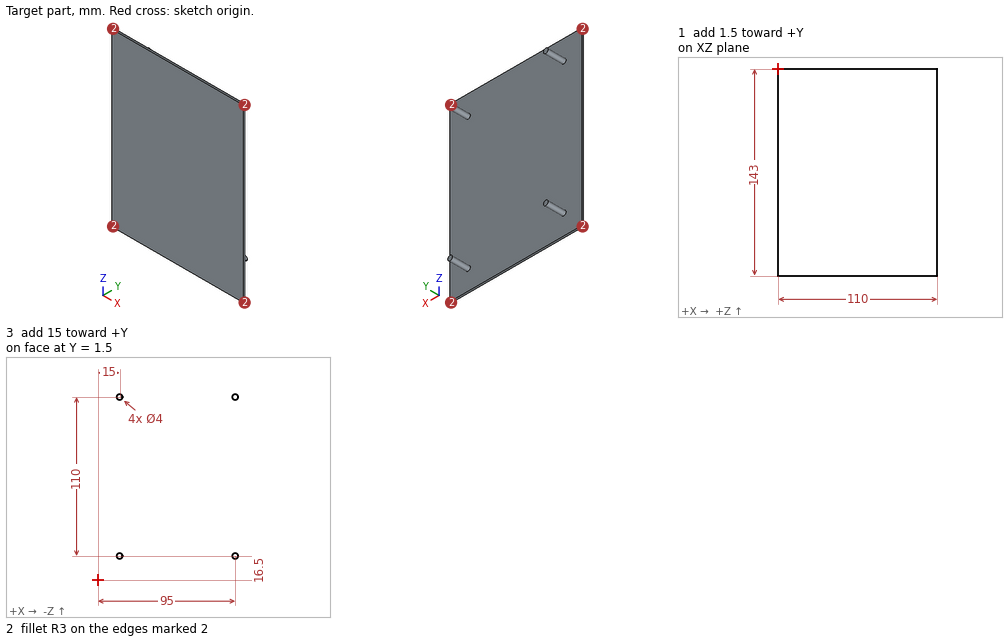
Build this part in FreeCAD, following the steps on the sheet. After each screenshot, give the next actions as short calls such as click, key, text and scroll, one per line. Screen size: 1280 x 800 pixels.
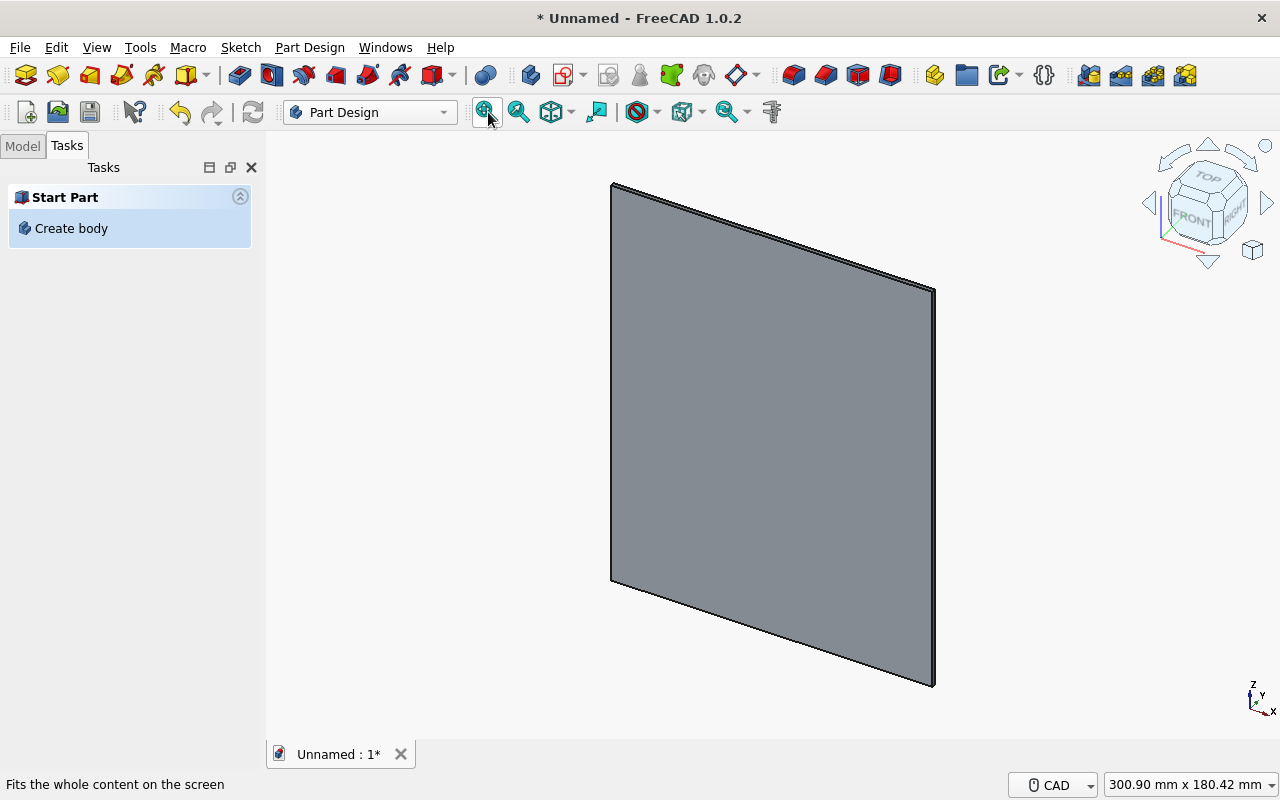
key(0)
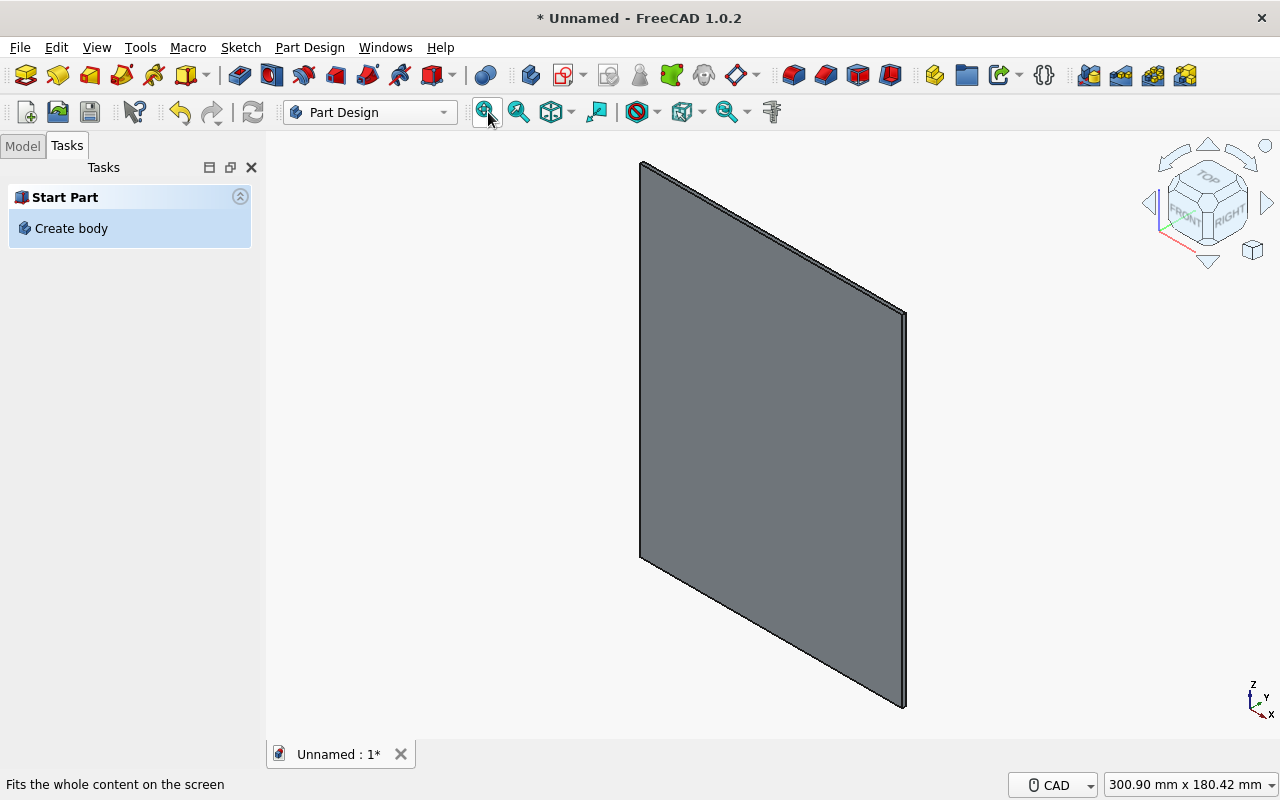
scroll(642, 555, up, 11)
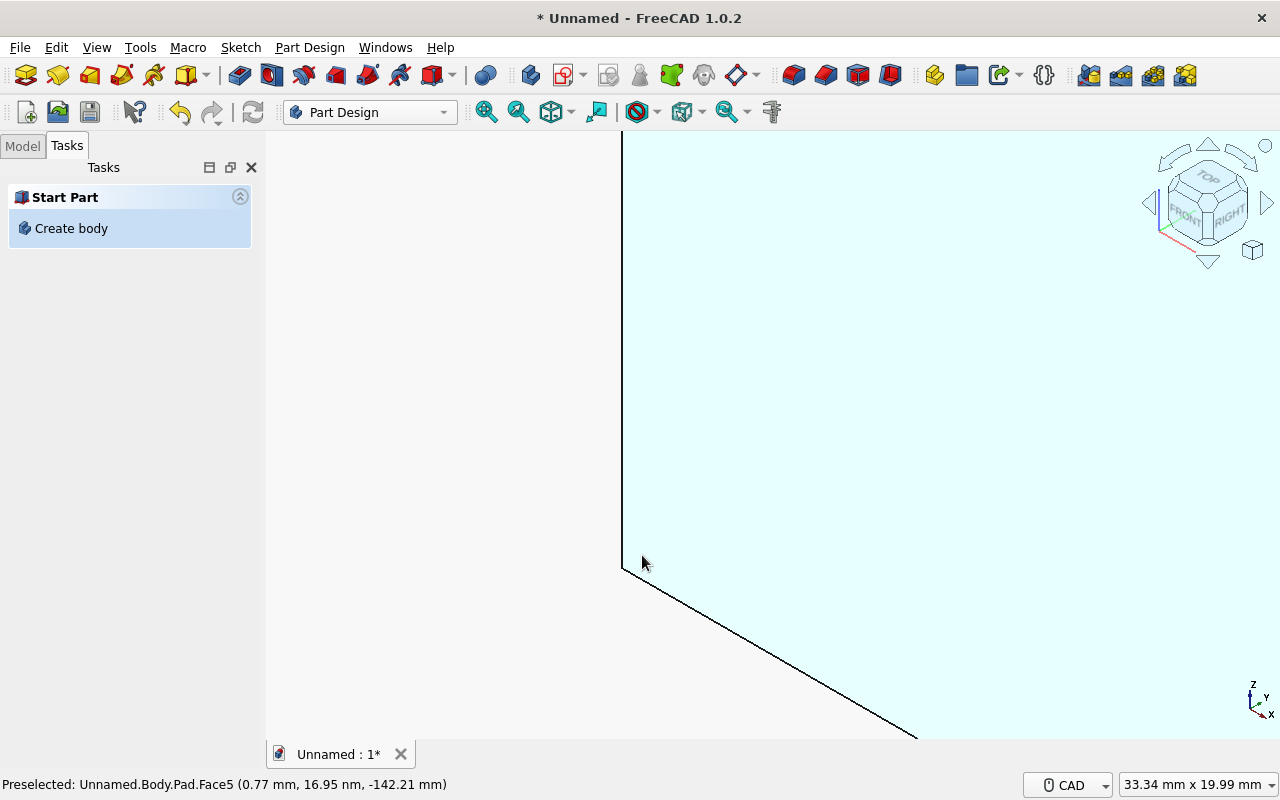
click(488, 112)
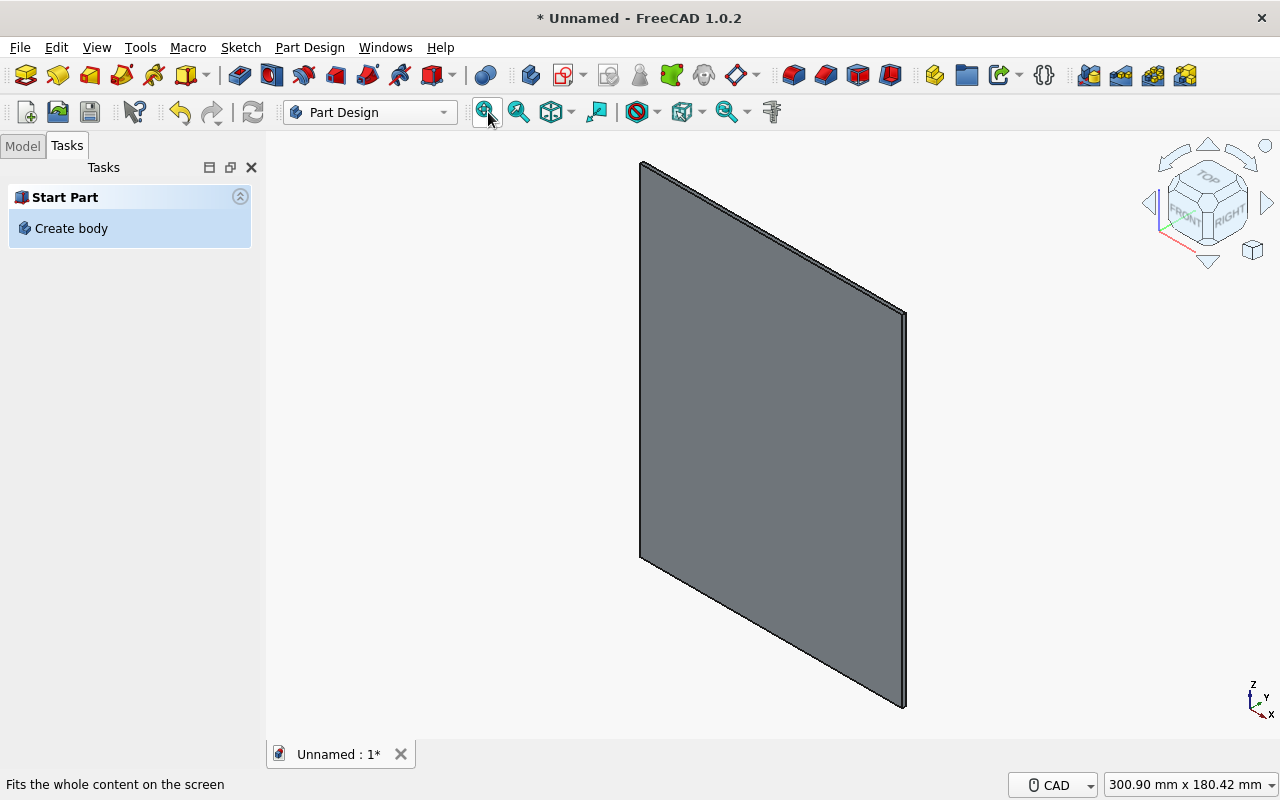
key(2)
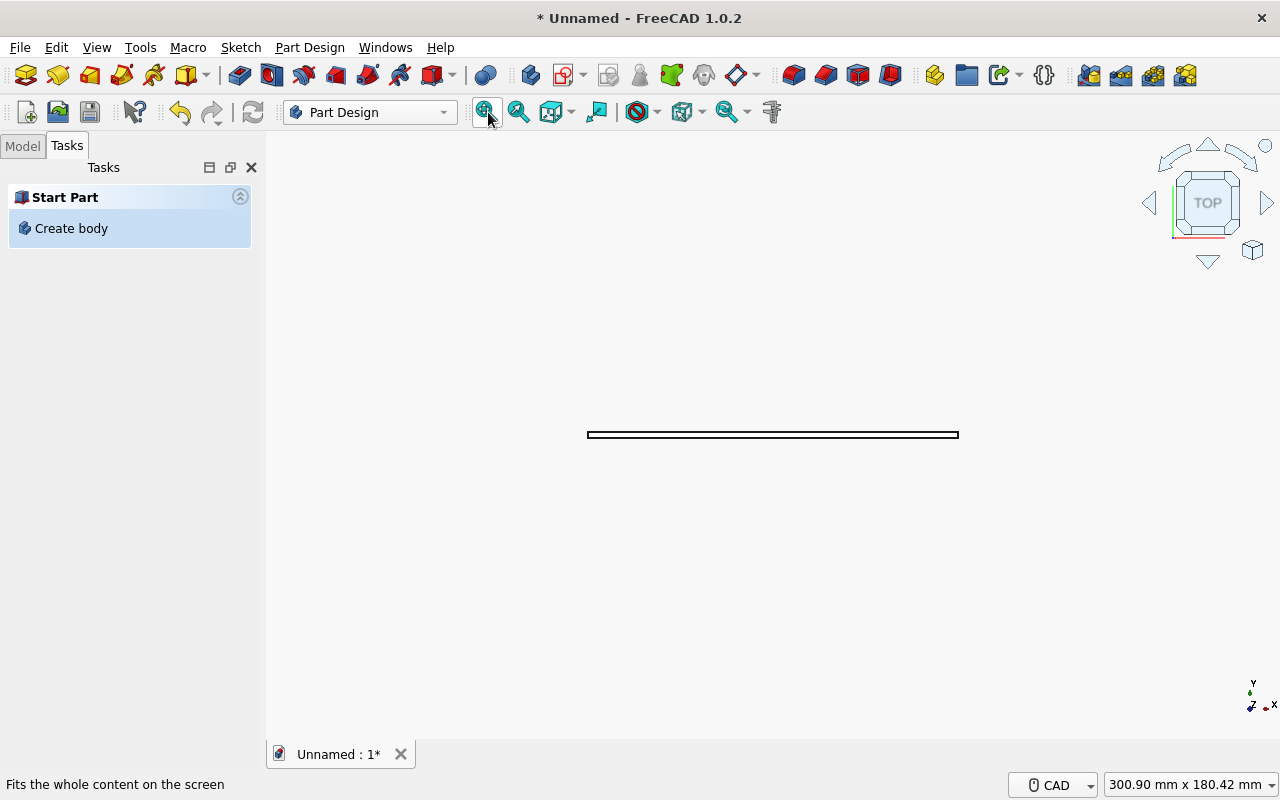
click(488, 112)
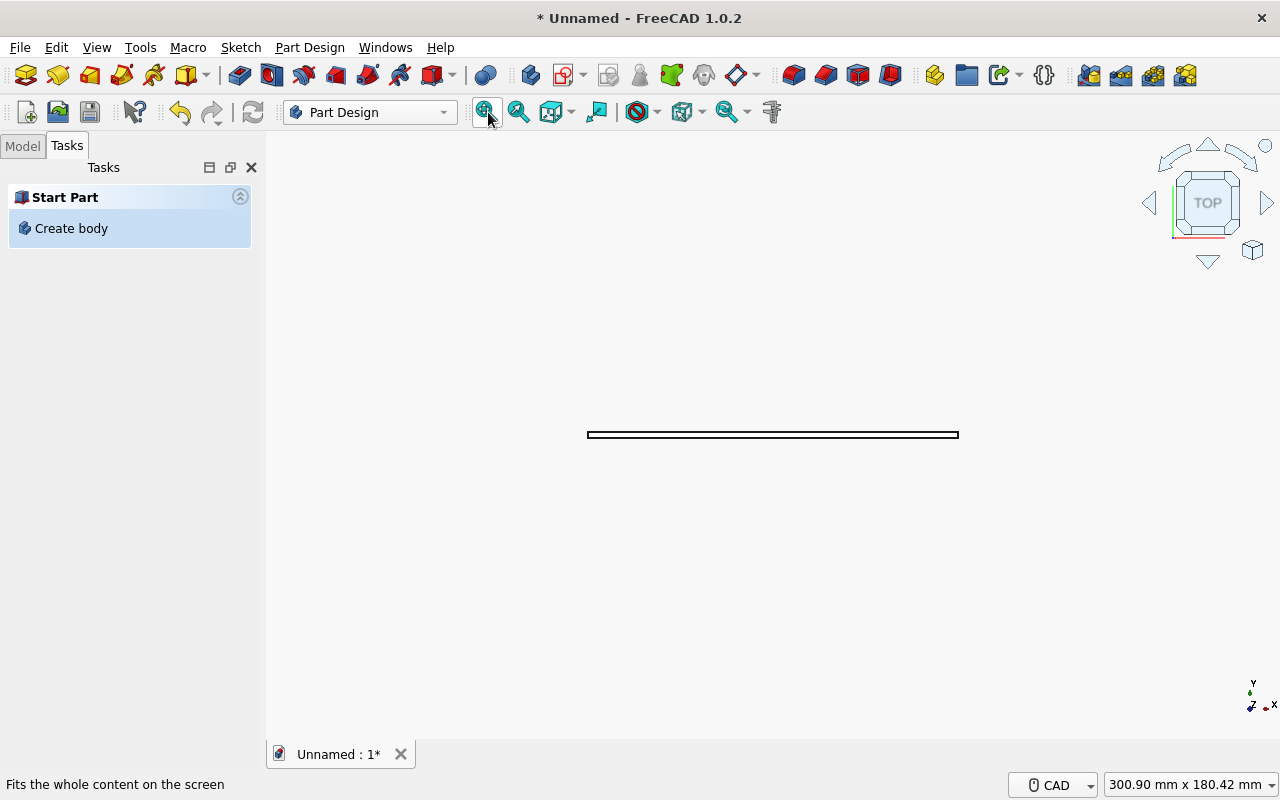
scroll(588, 434, up, 11)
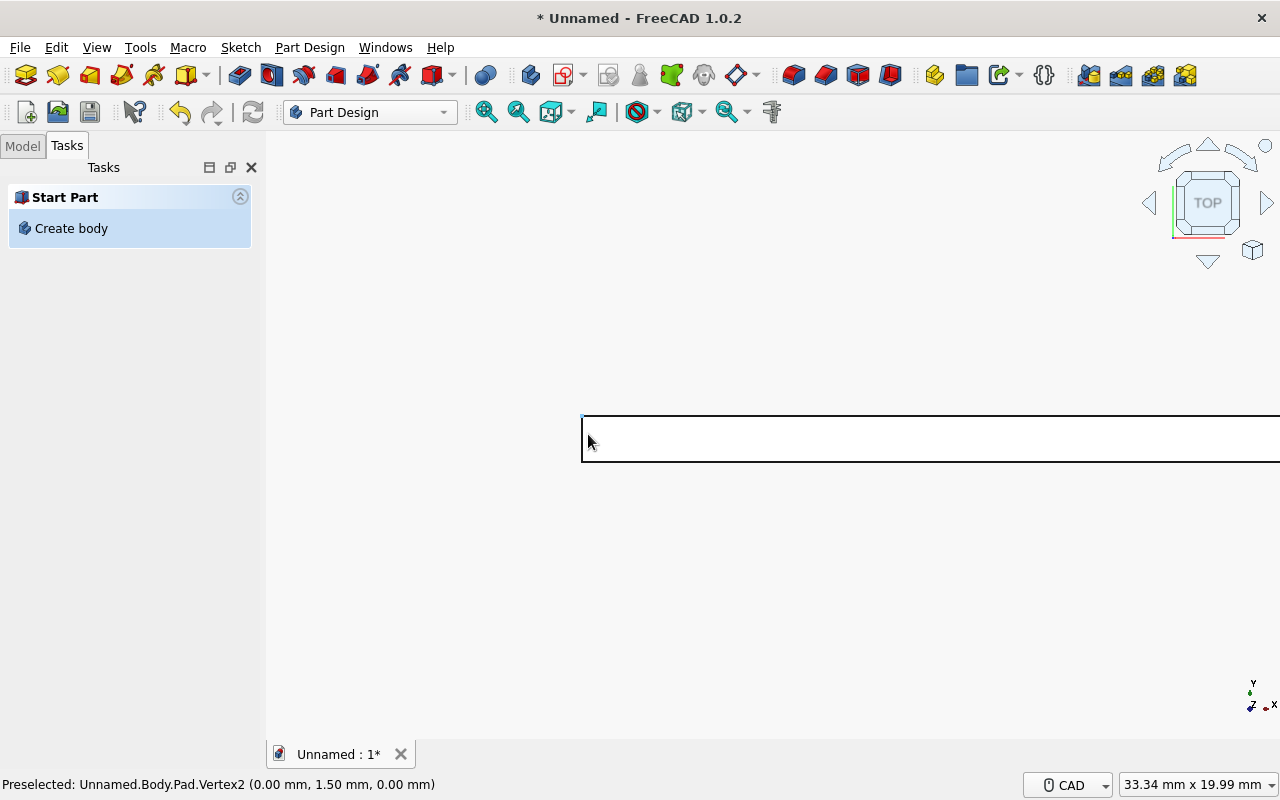
click(582, 438)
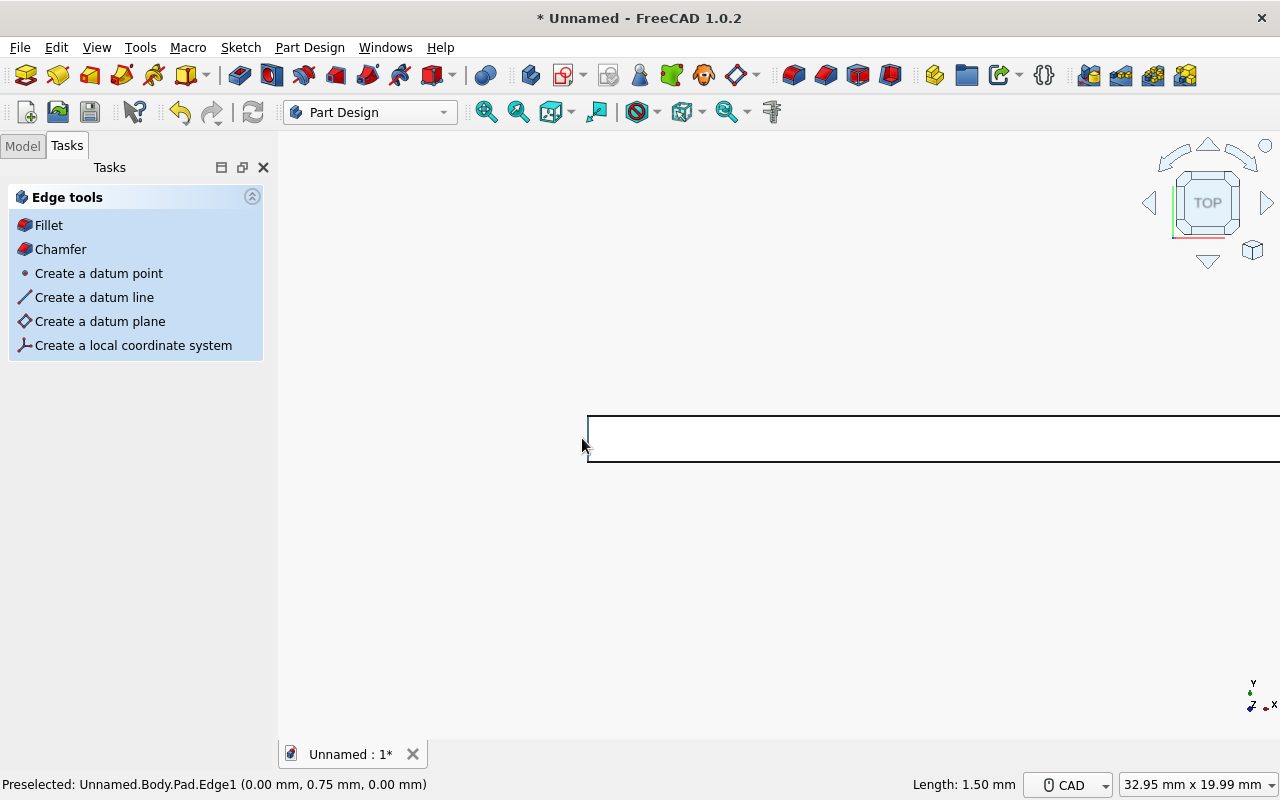
click(488, 112)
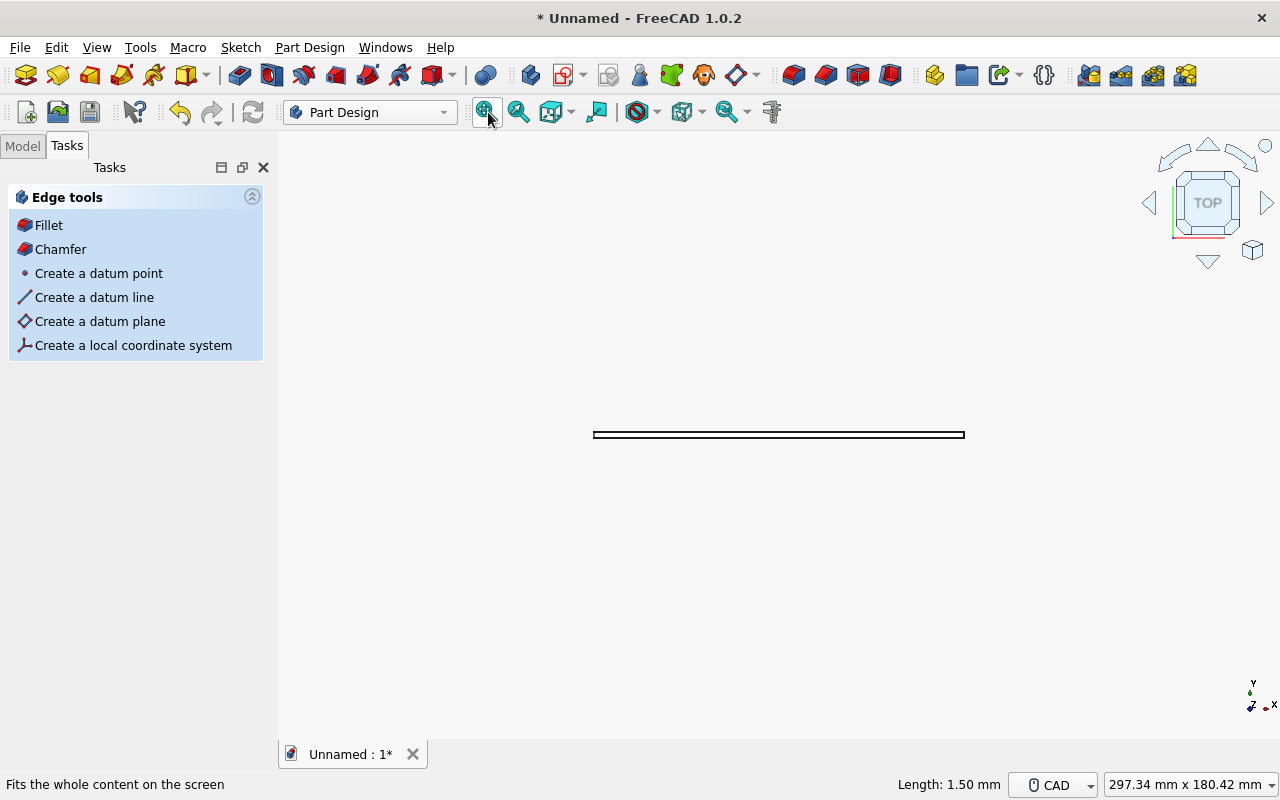
key(1)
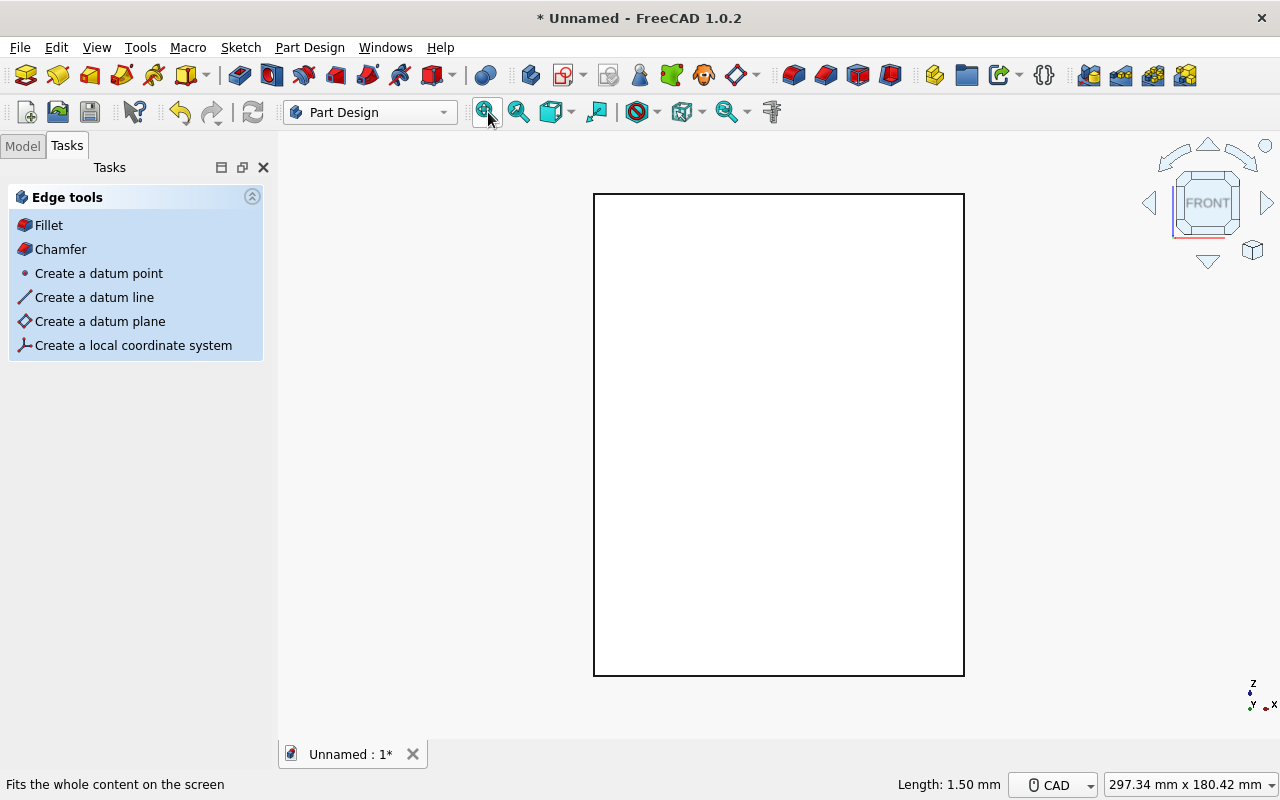
scroll(594, 675, up, 11)